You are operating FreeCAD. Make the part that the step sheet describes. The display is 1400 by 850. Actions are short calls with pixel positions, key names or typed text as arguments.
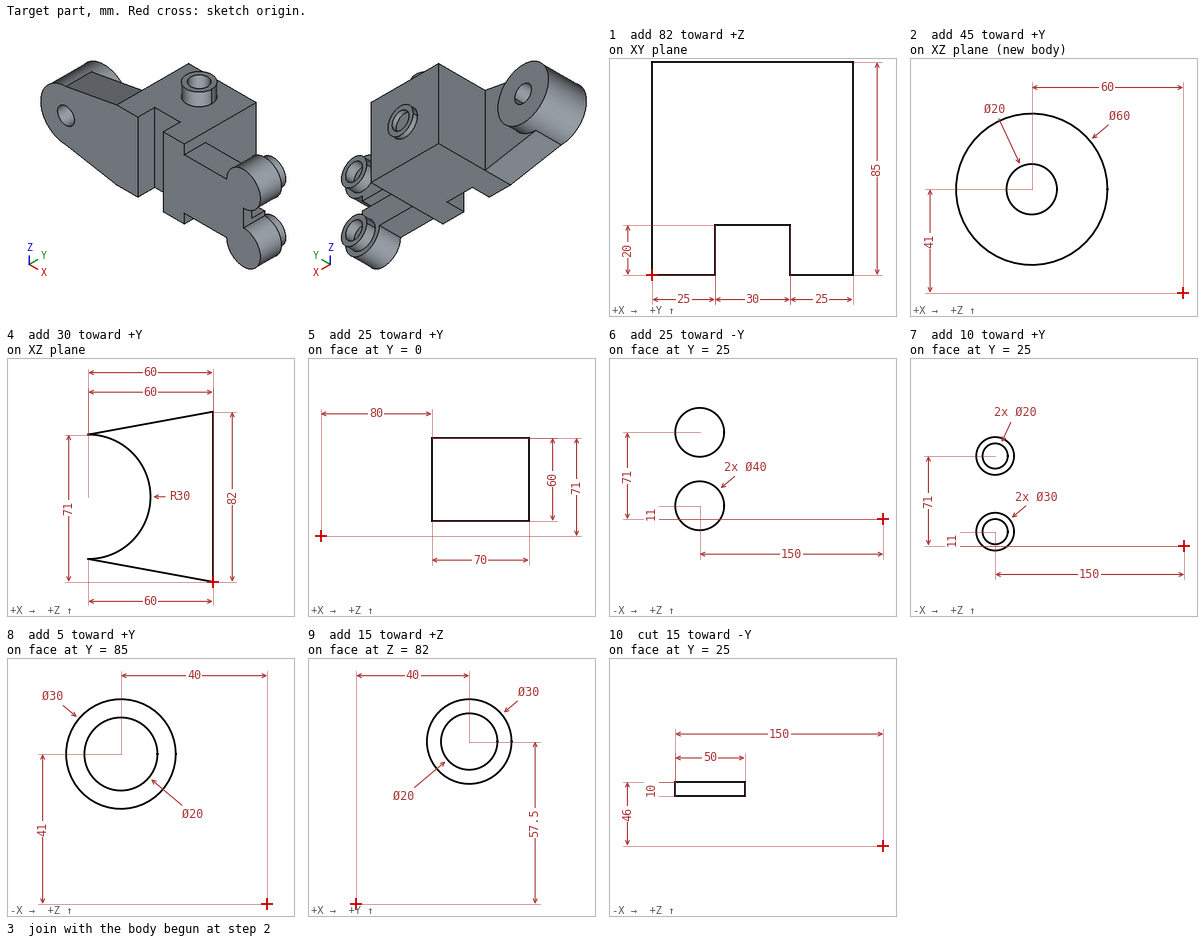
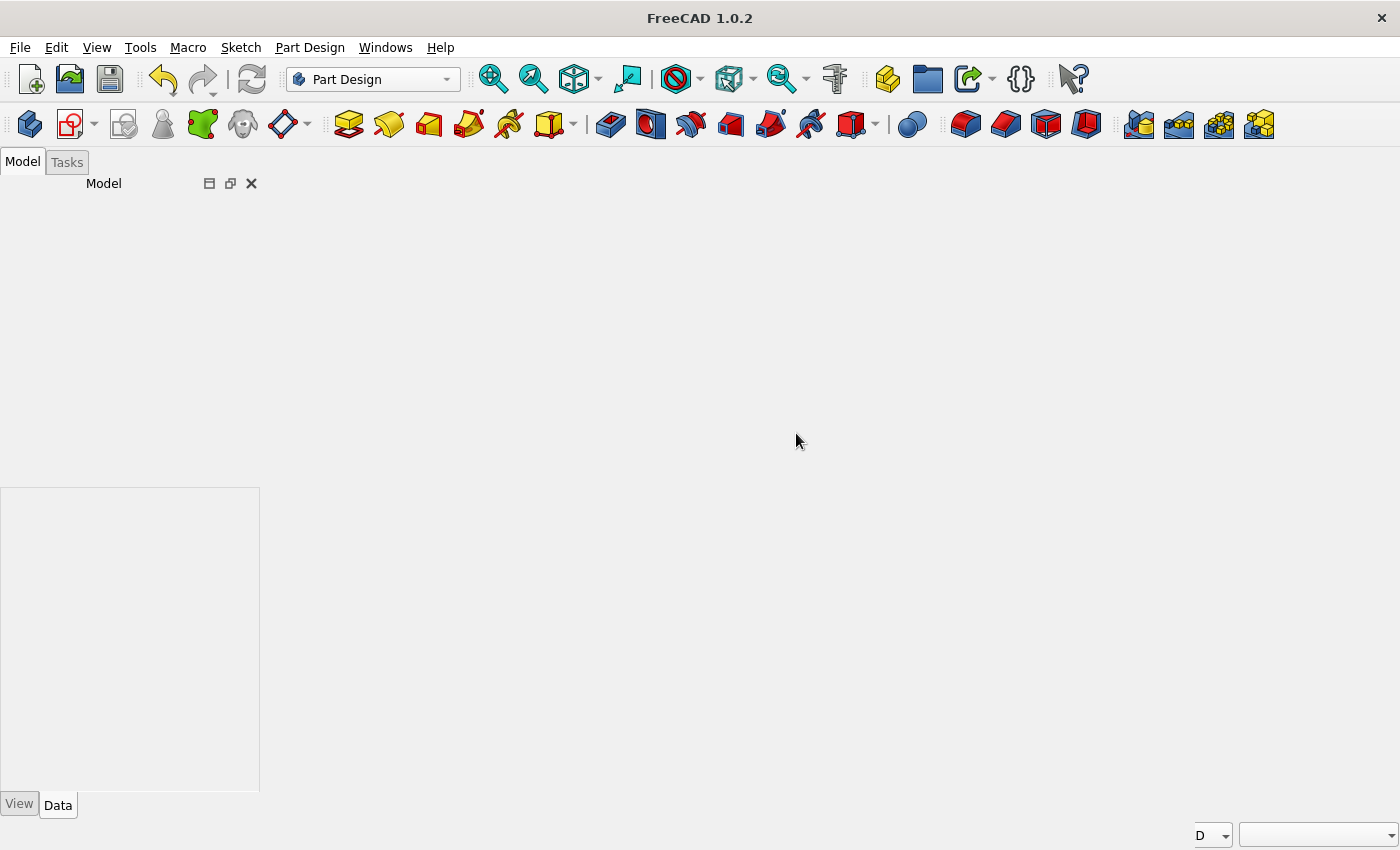
click(30, 80)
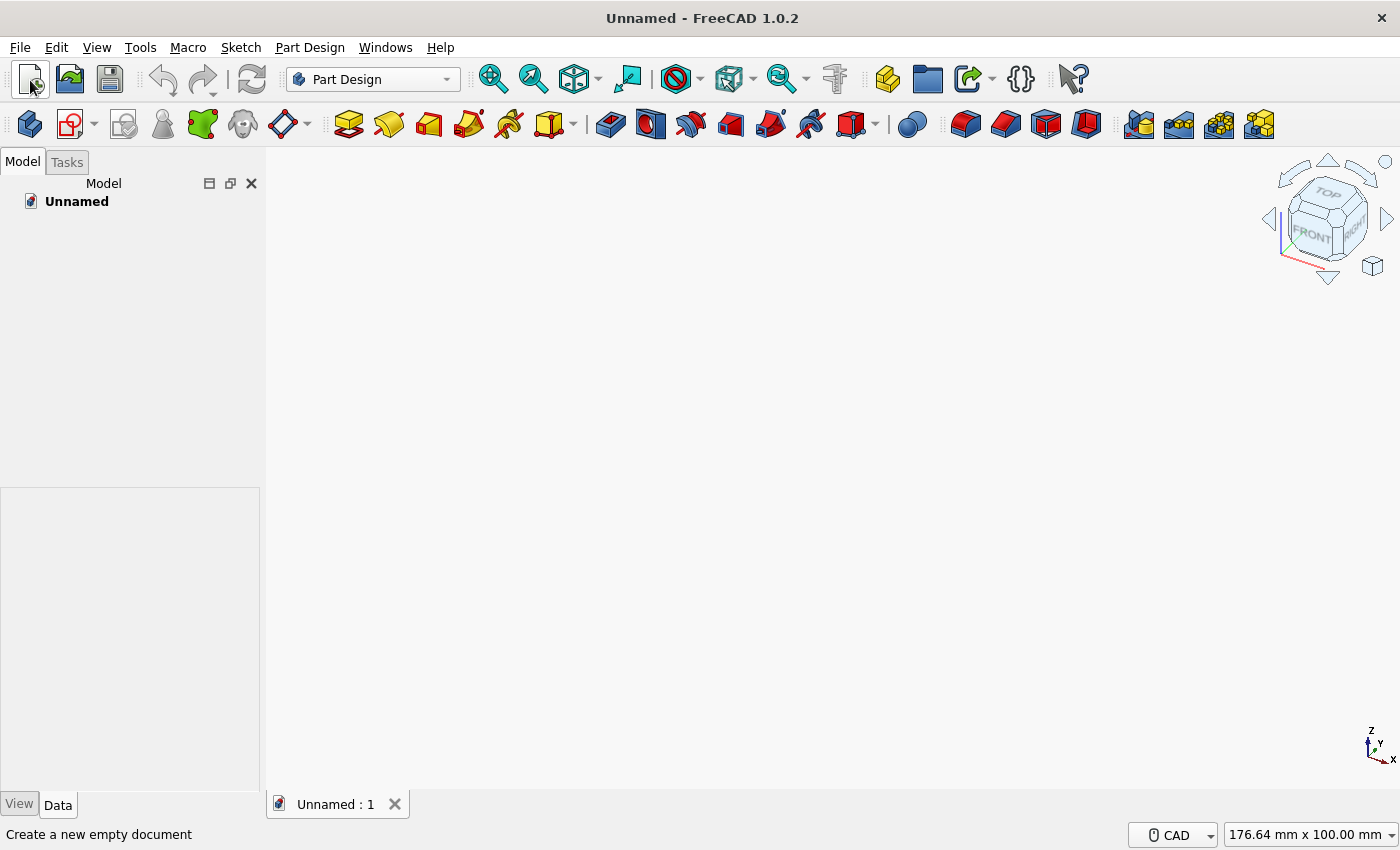
click(70, 124)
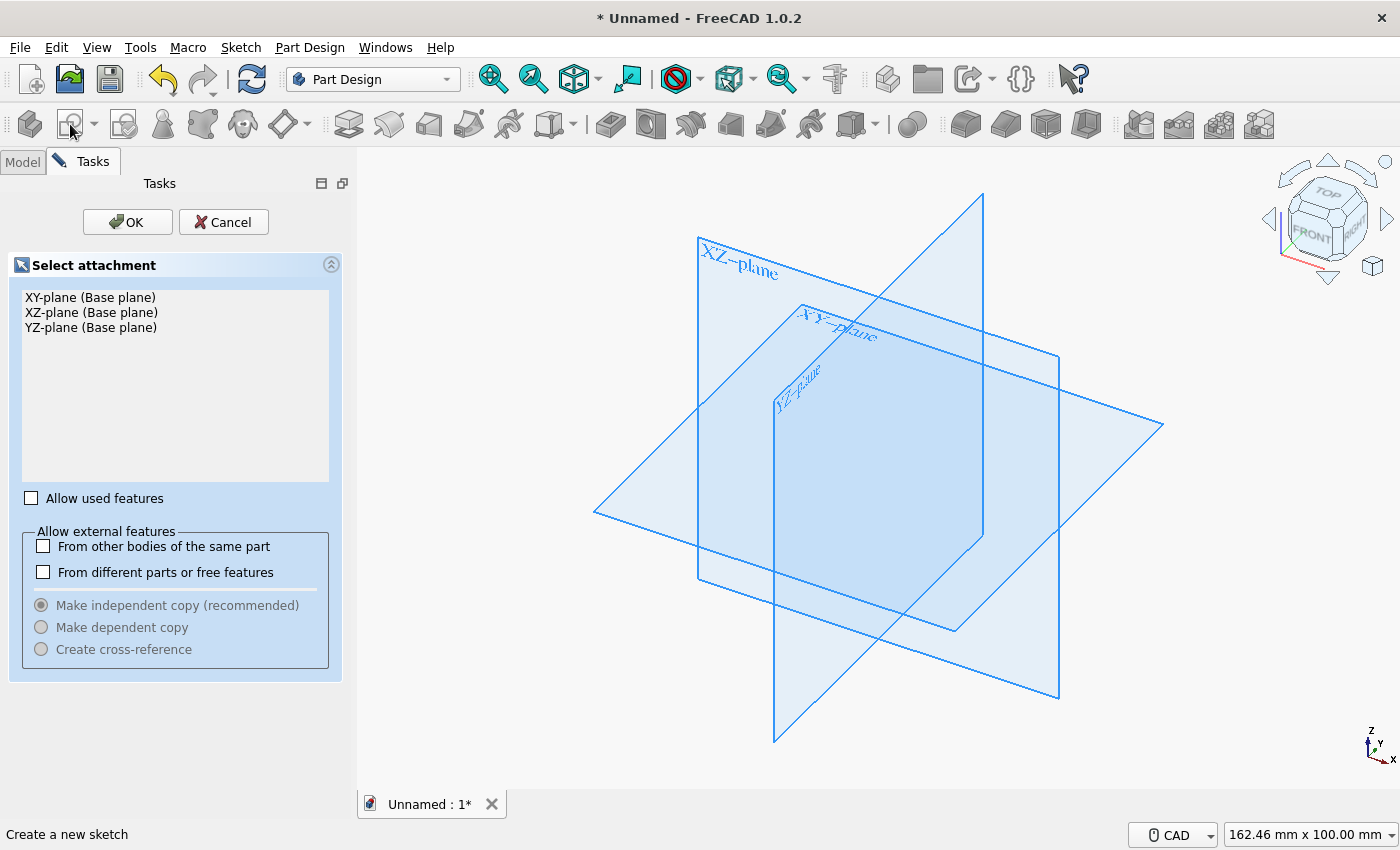
click(82, 298)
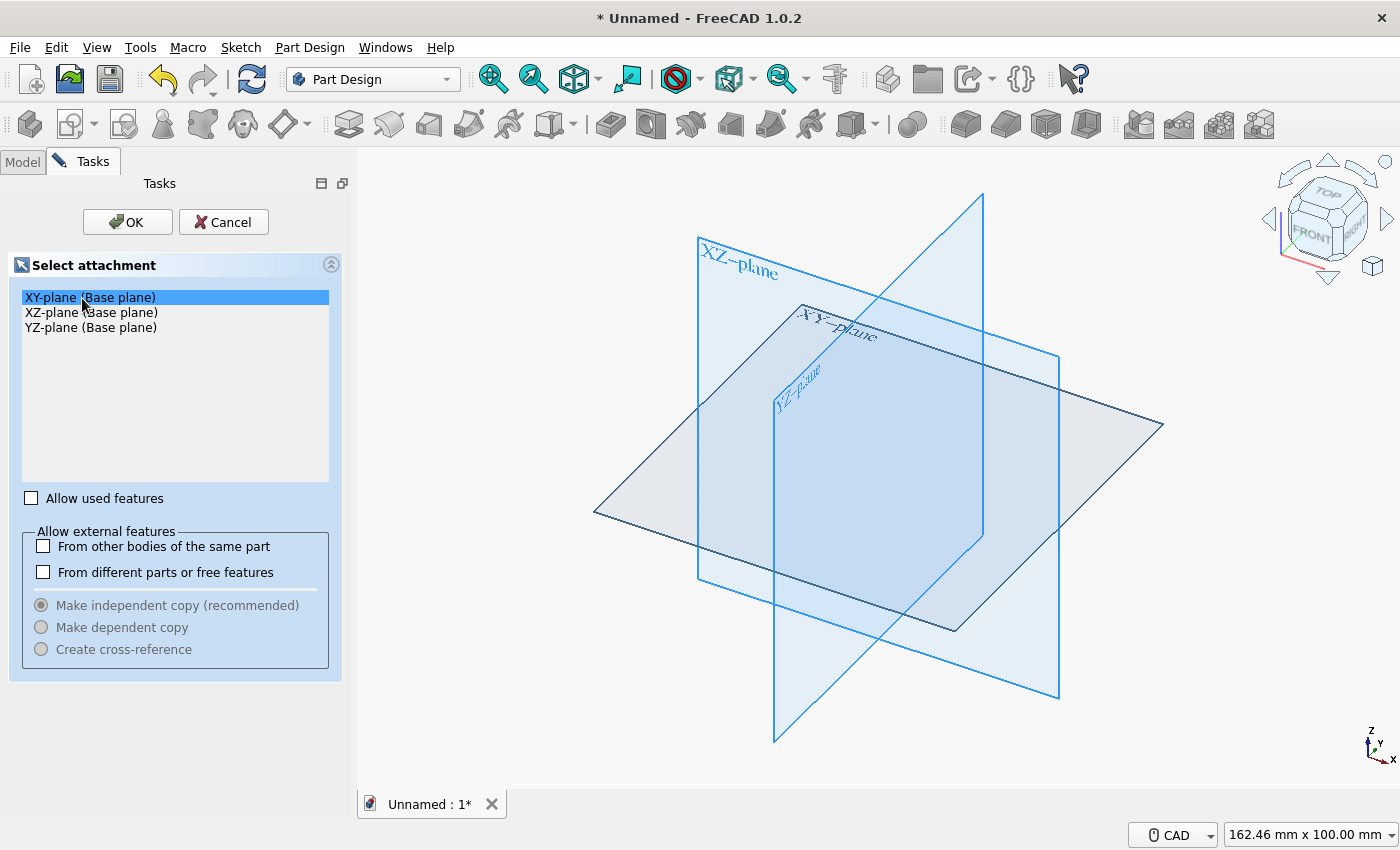
click(128, 222)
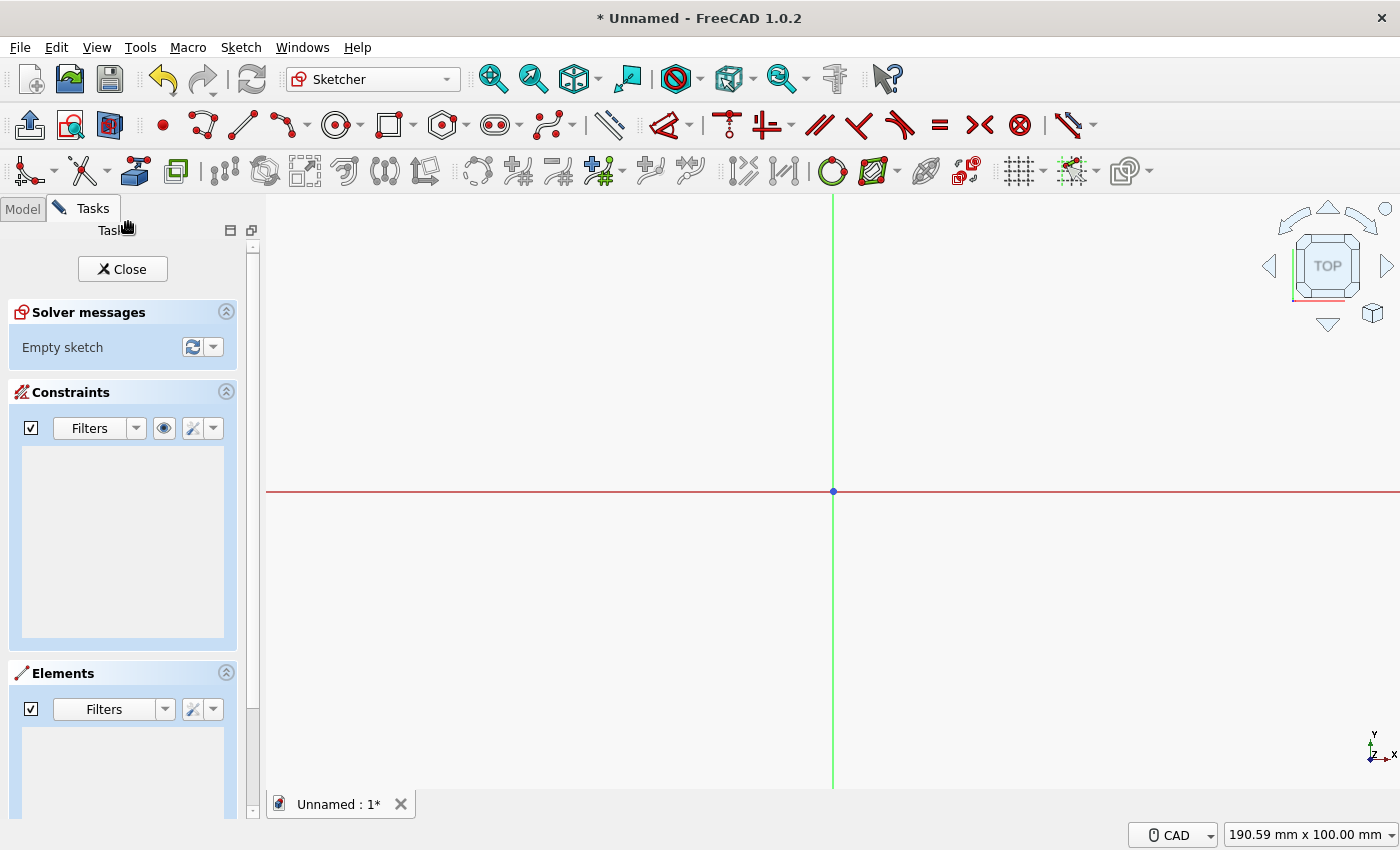
scroll(392, 761, down, 3)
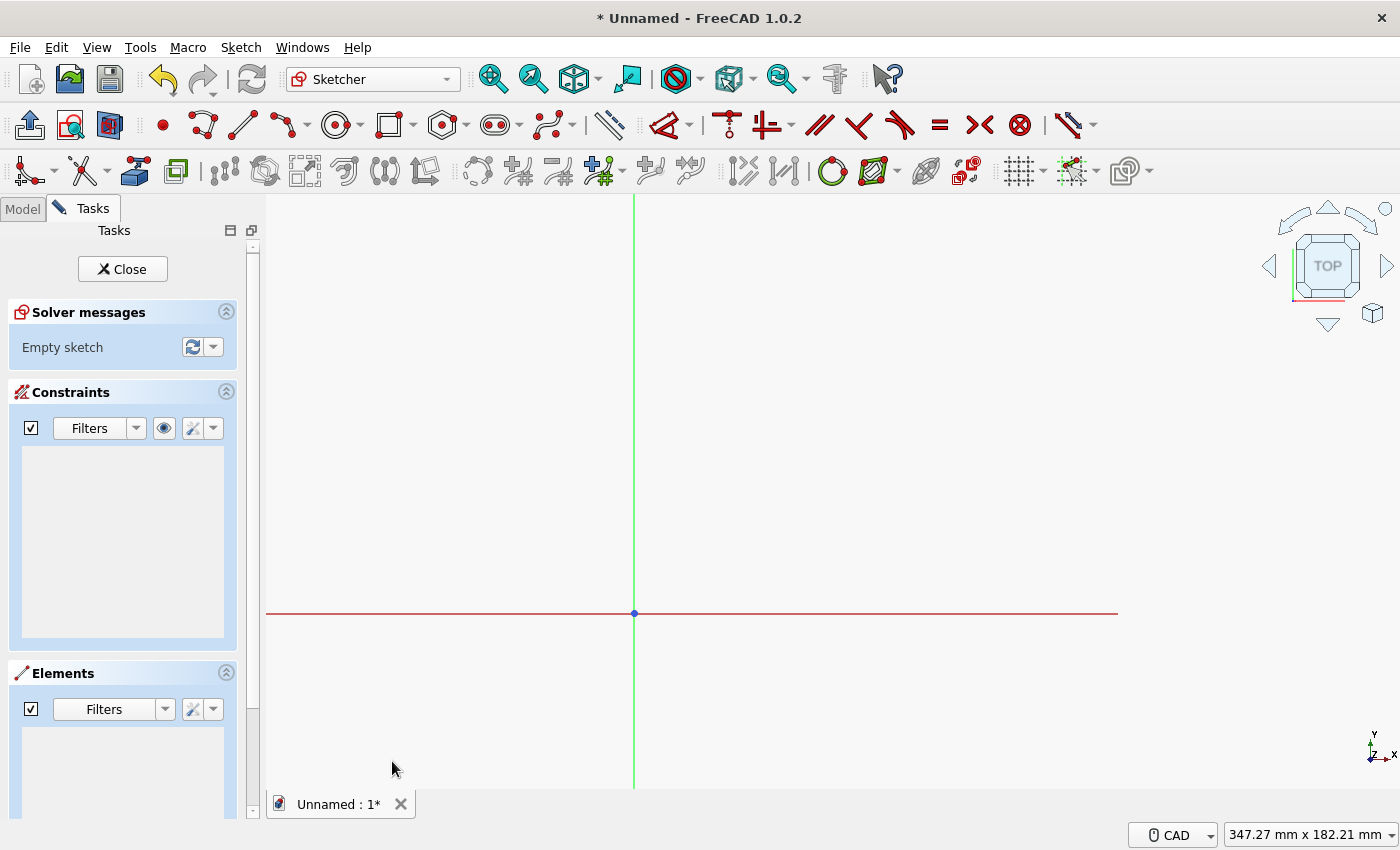
scroll(765, 441, up, 2)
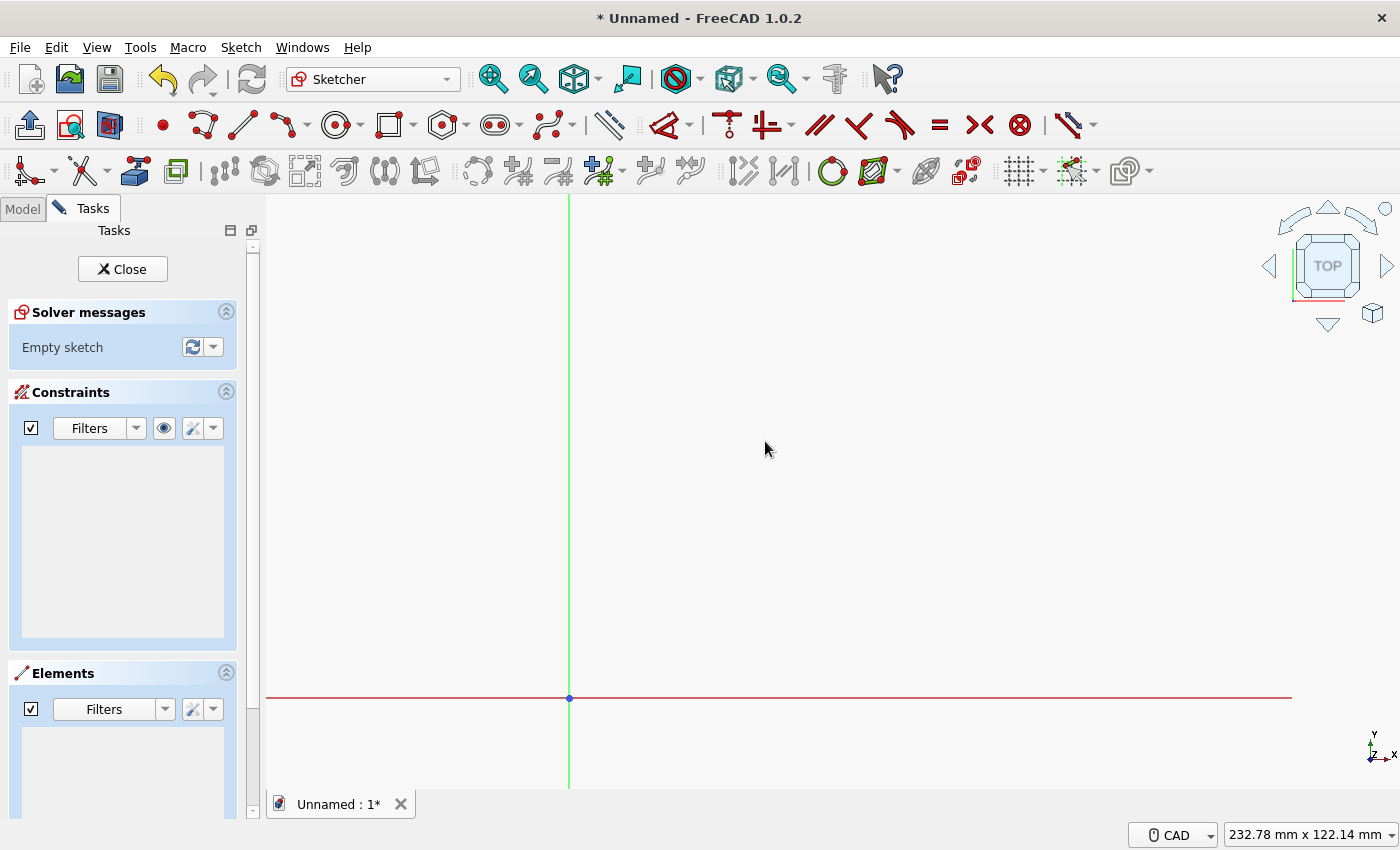
click(204, 126)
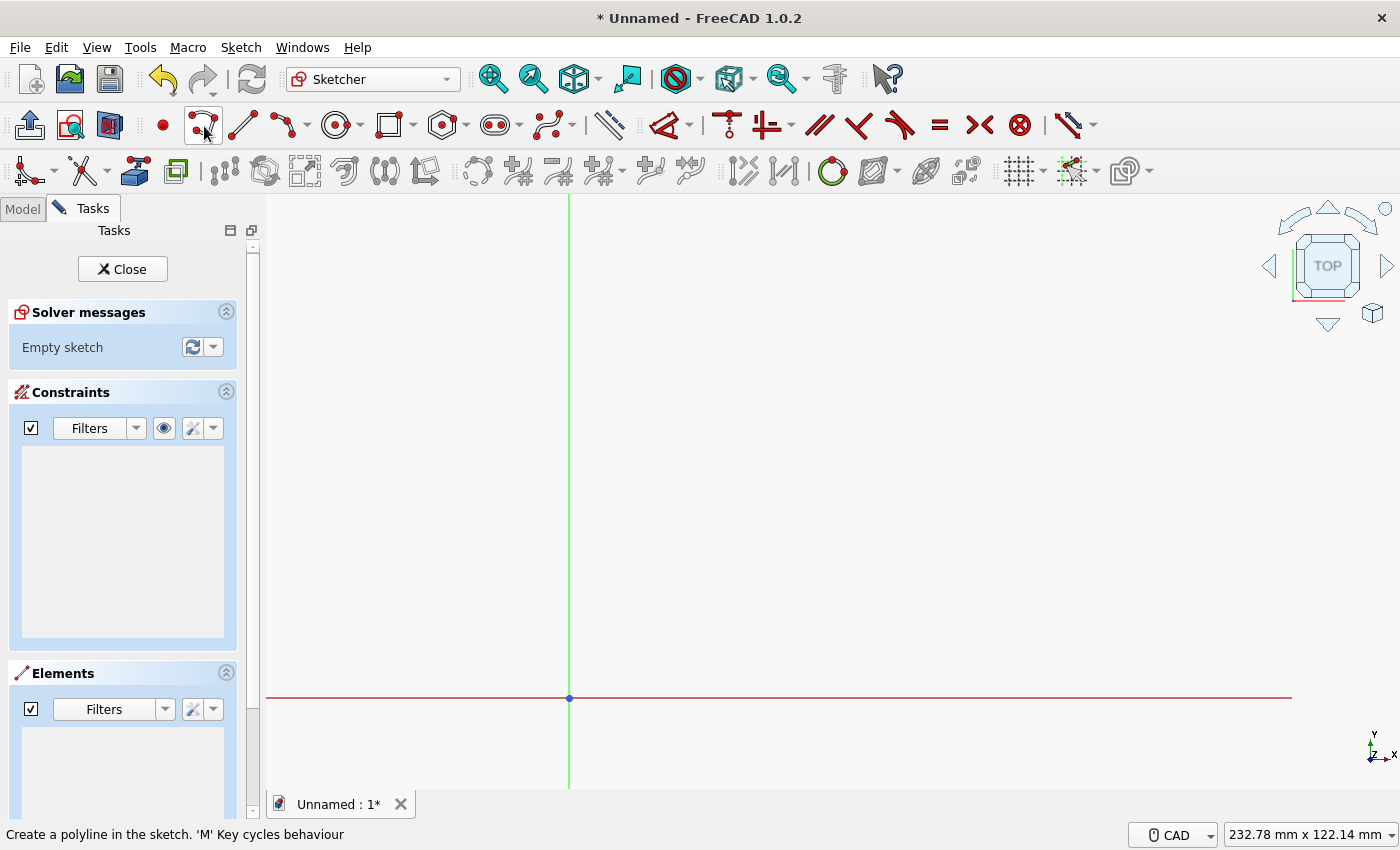
click(569, 698)
click(691, 689)
click(691, 601)
click(837, 601)
click(837, 698)
click(959, 689)
click(959, 284)
click(578, 284)
click(569, 698)
key(Escape)
key(Escape)